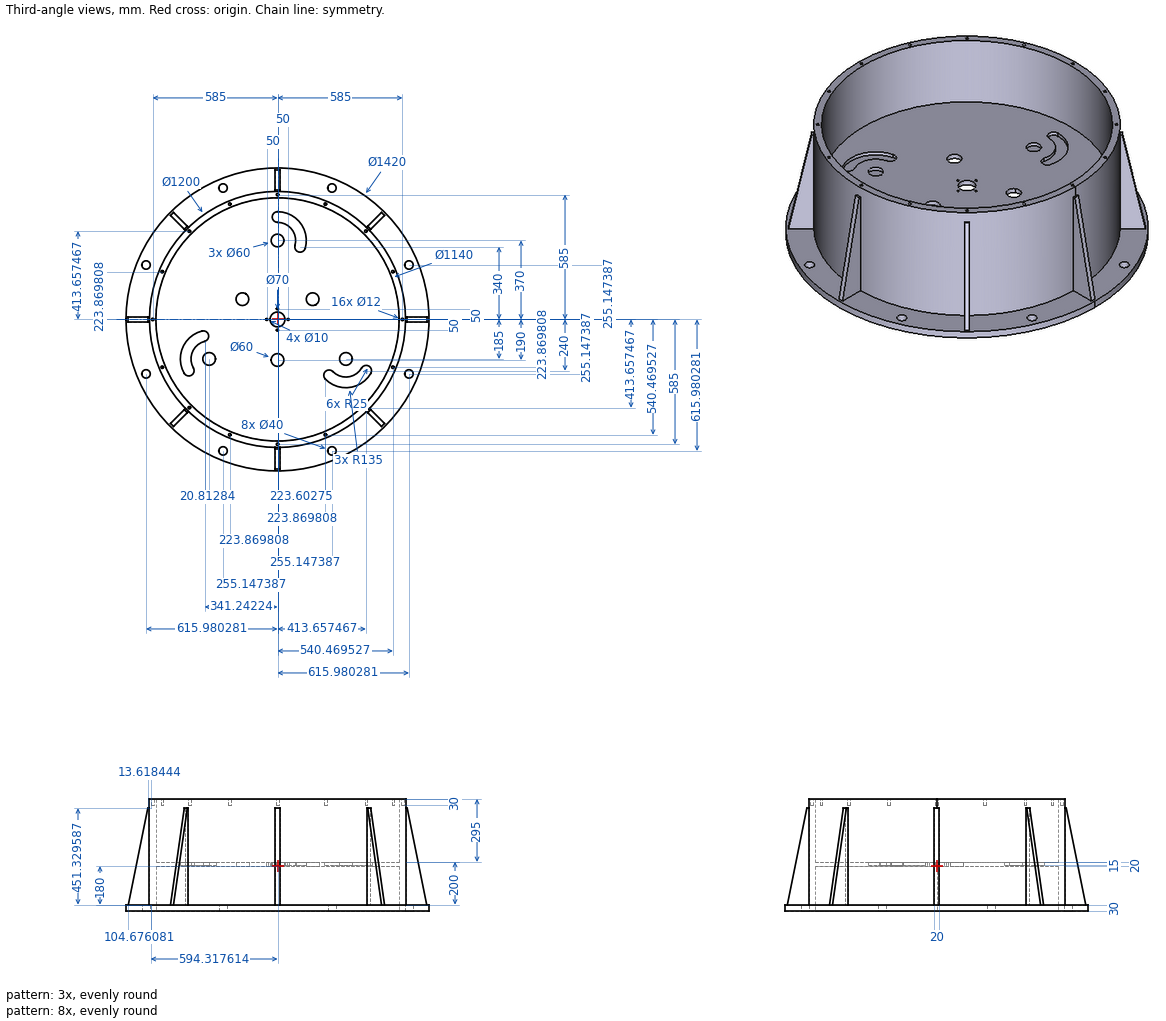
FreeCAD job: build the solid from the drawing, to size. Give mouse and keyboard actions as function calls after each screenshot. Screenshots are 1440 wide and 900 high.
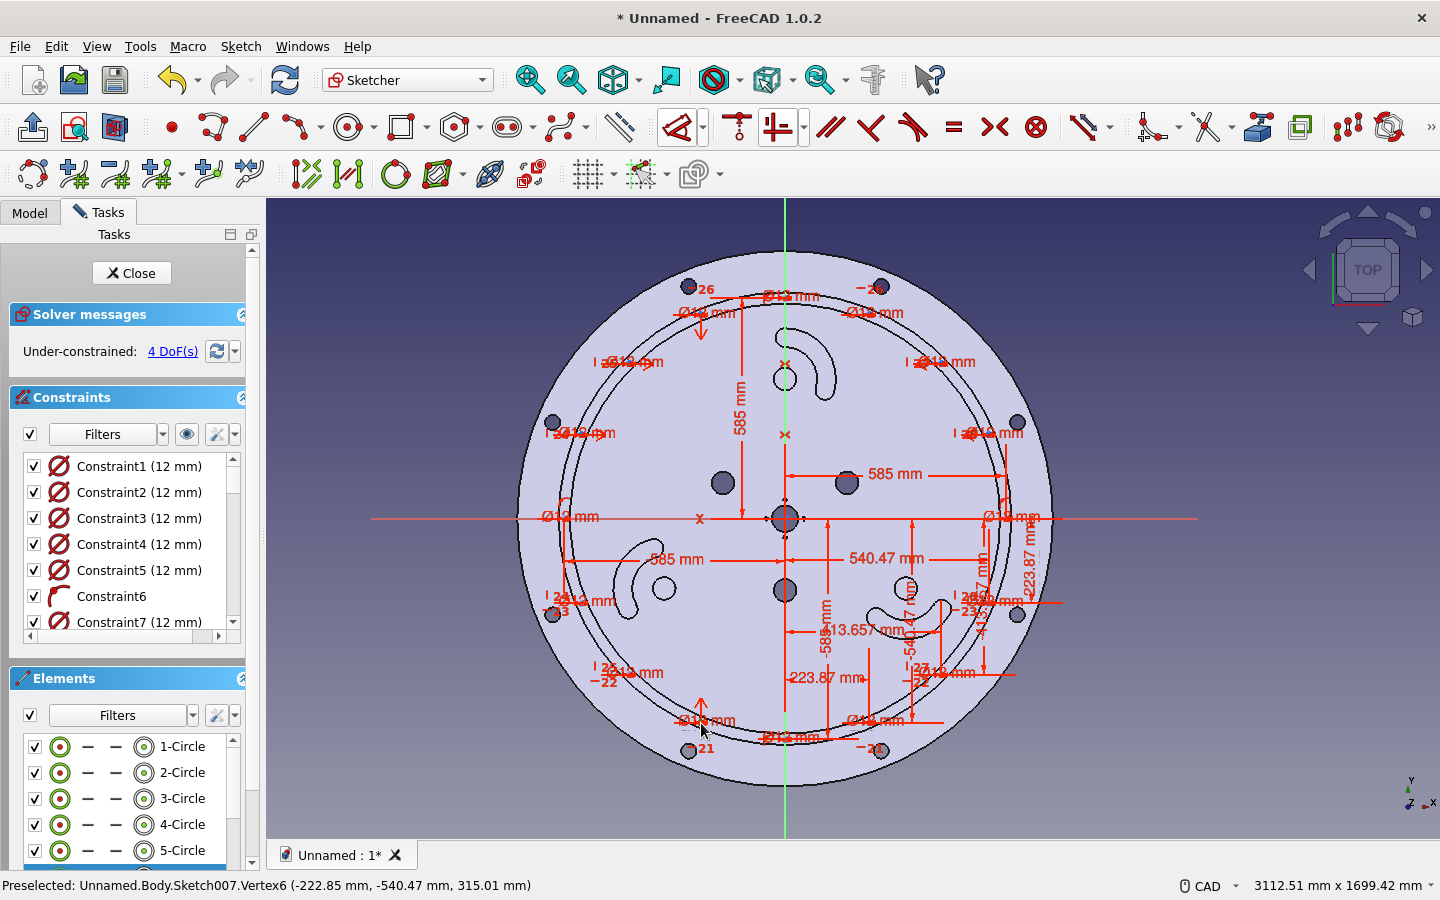
key(l)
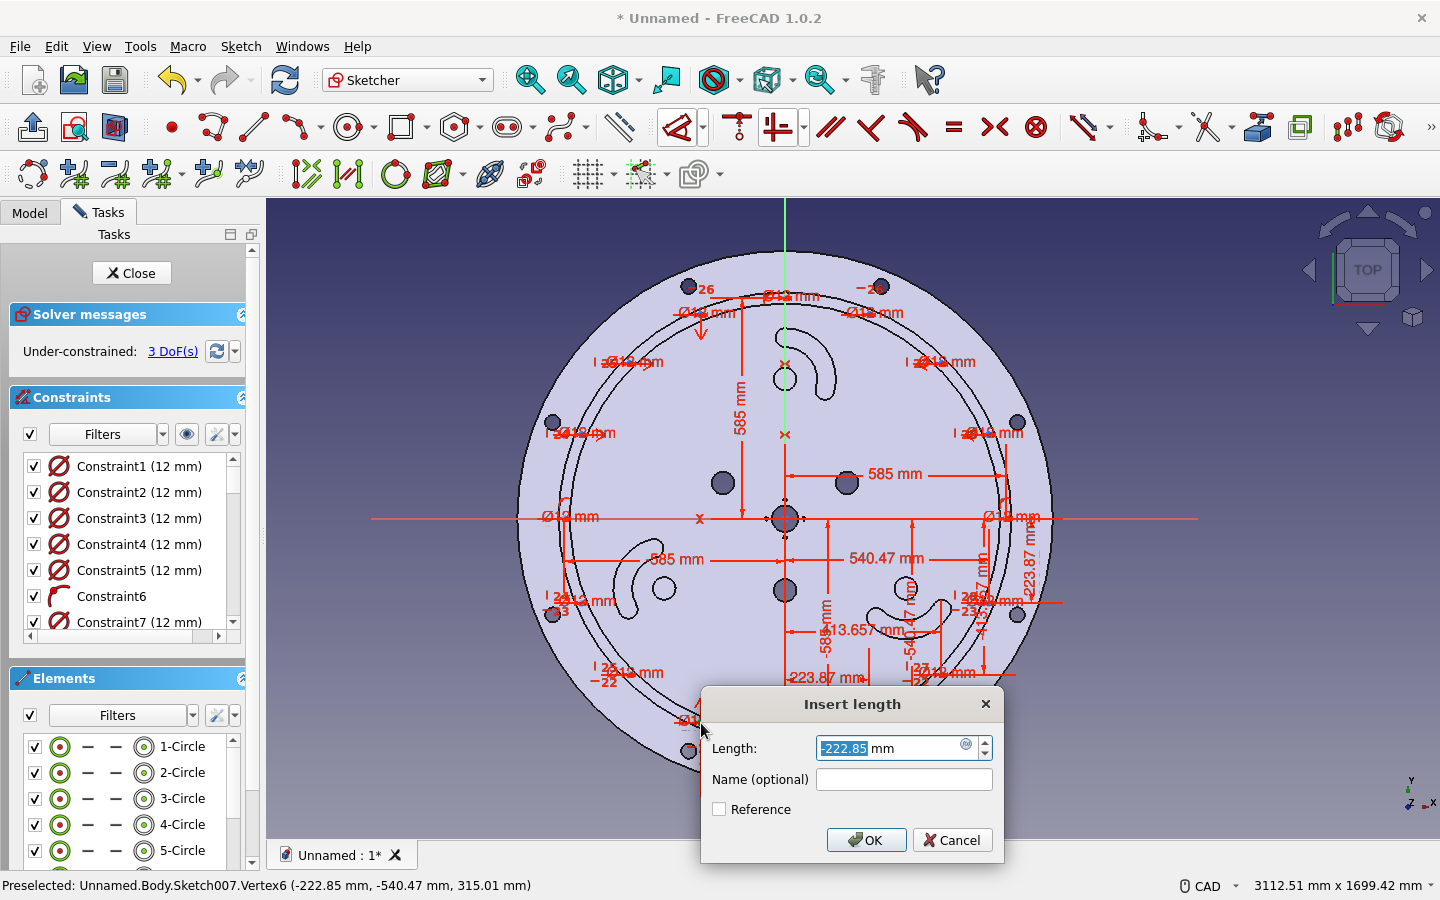
text(-223.869808)
key(Return)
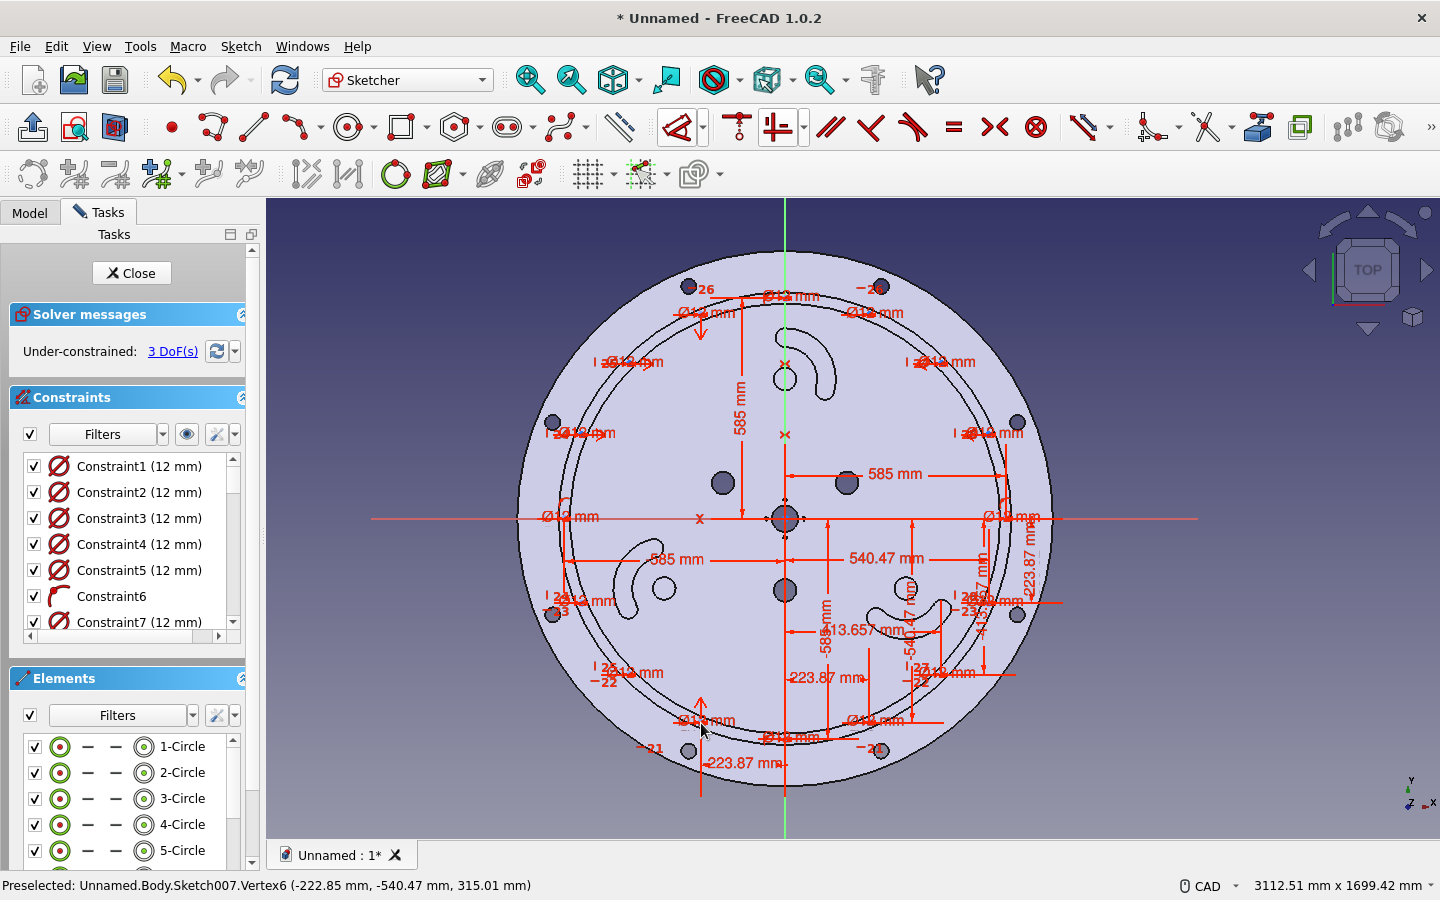
click(581, 435)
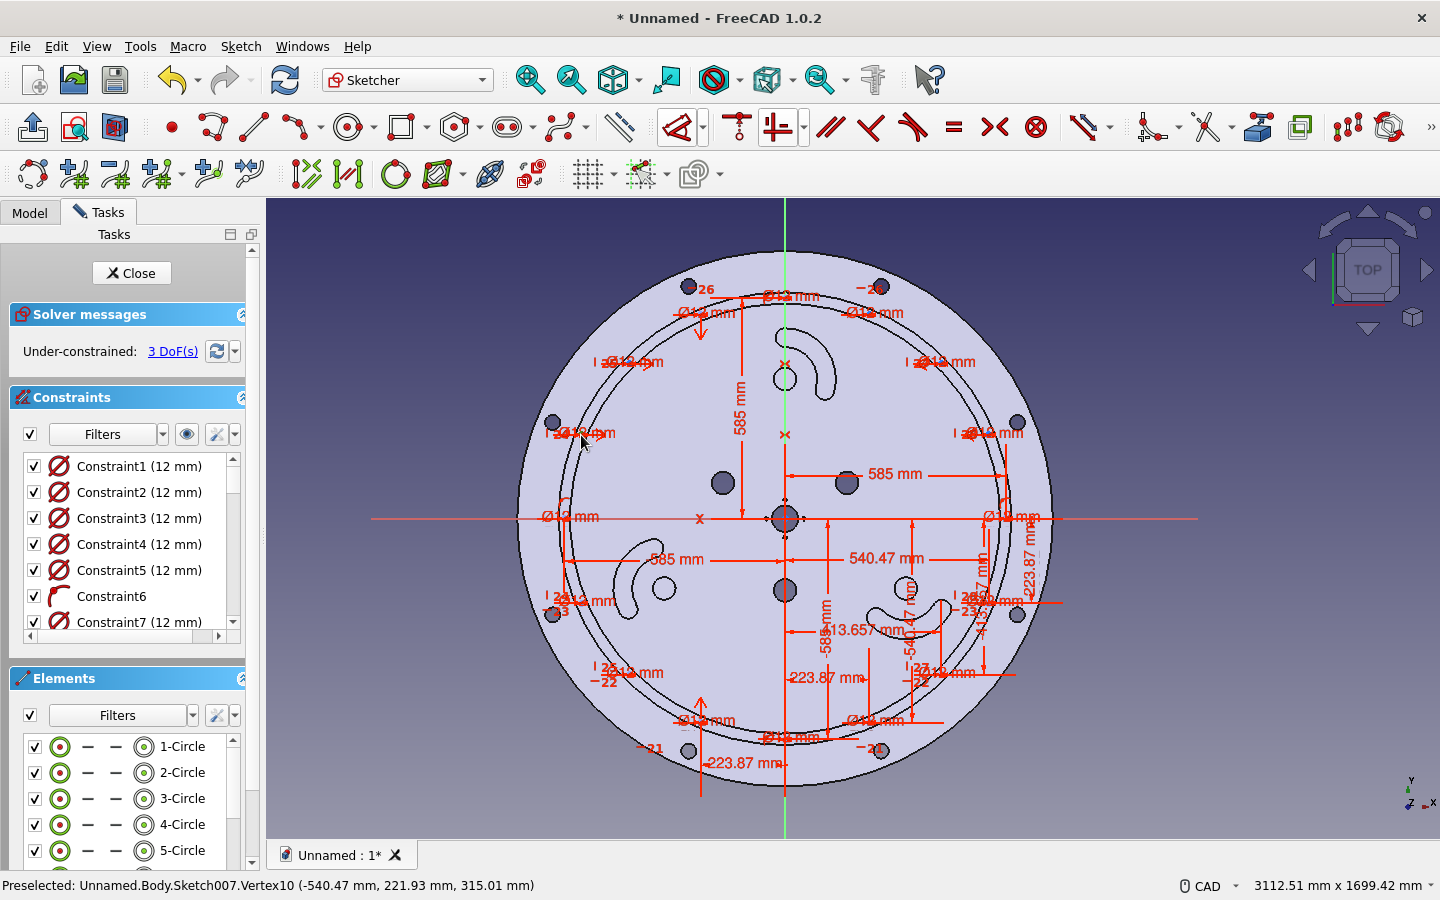
key(i)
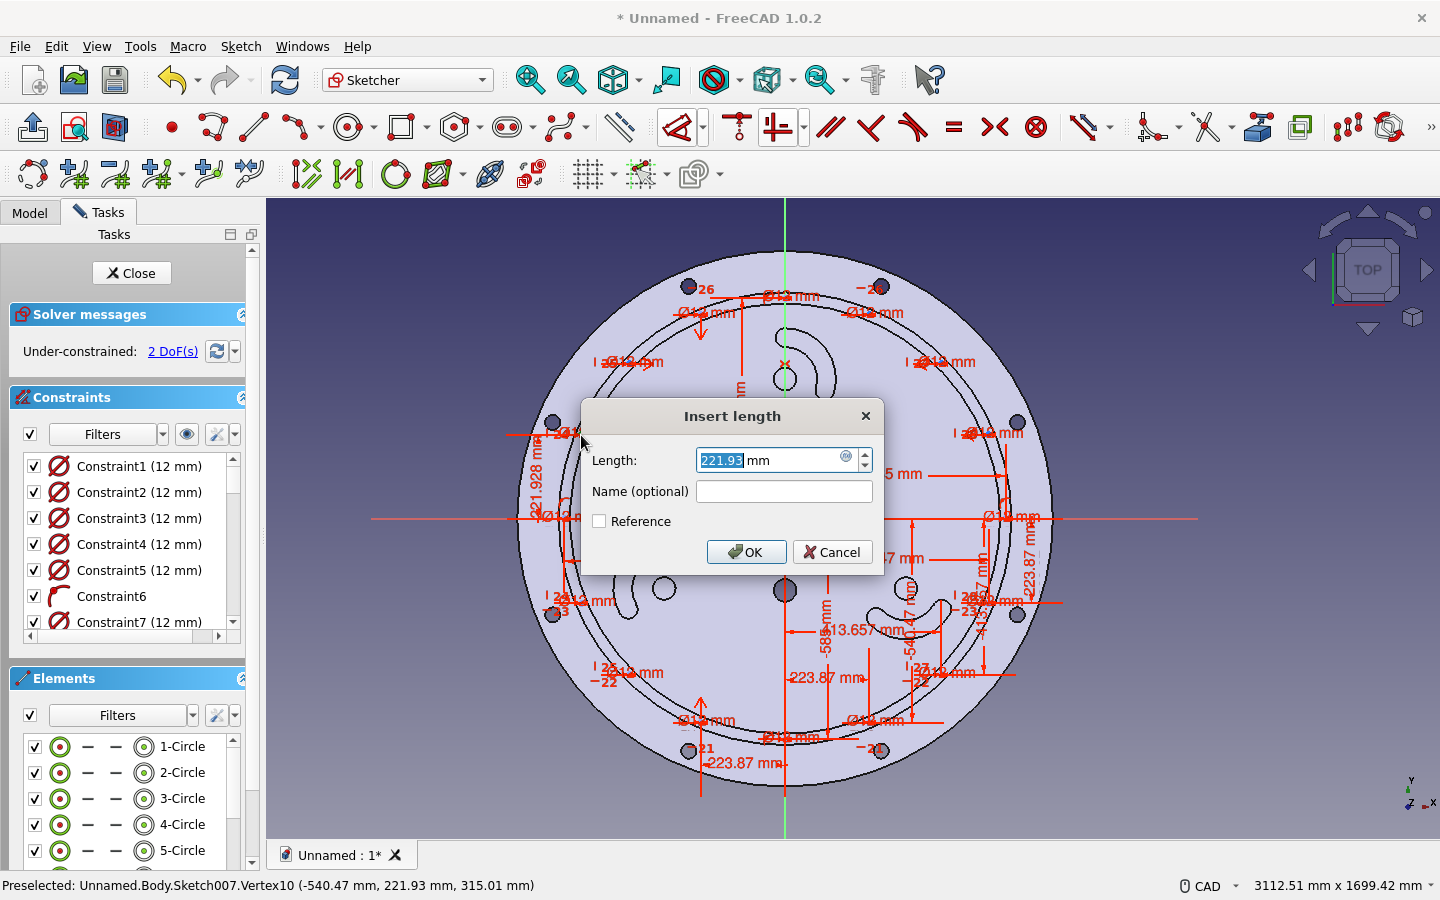
text(223.869808)
key(Return)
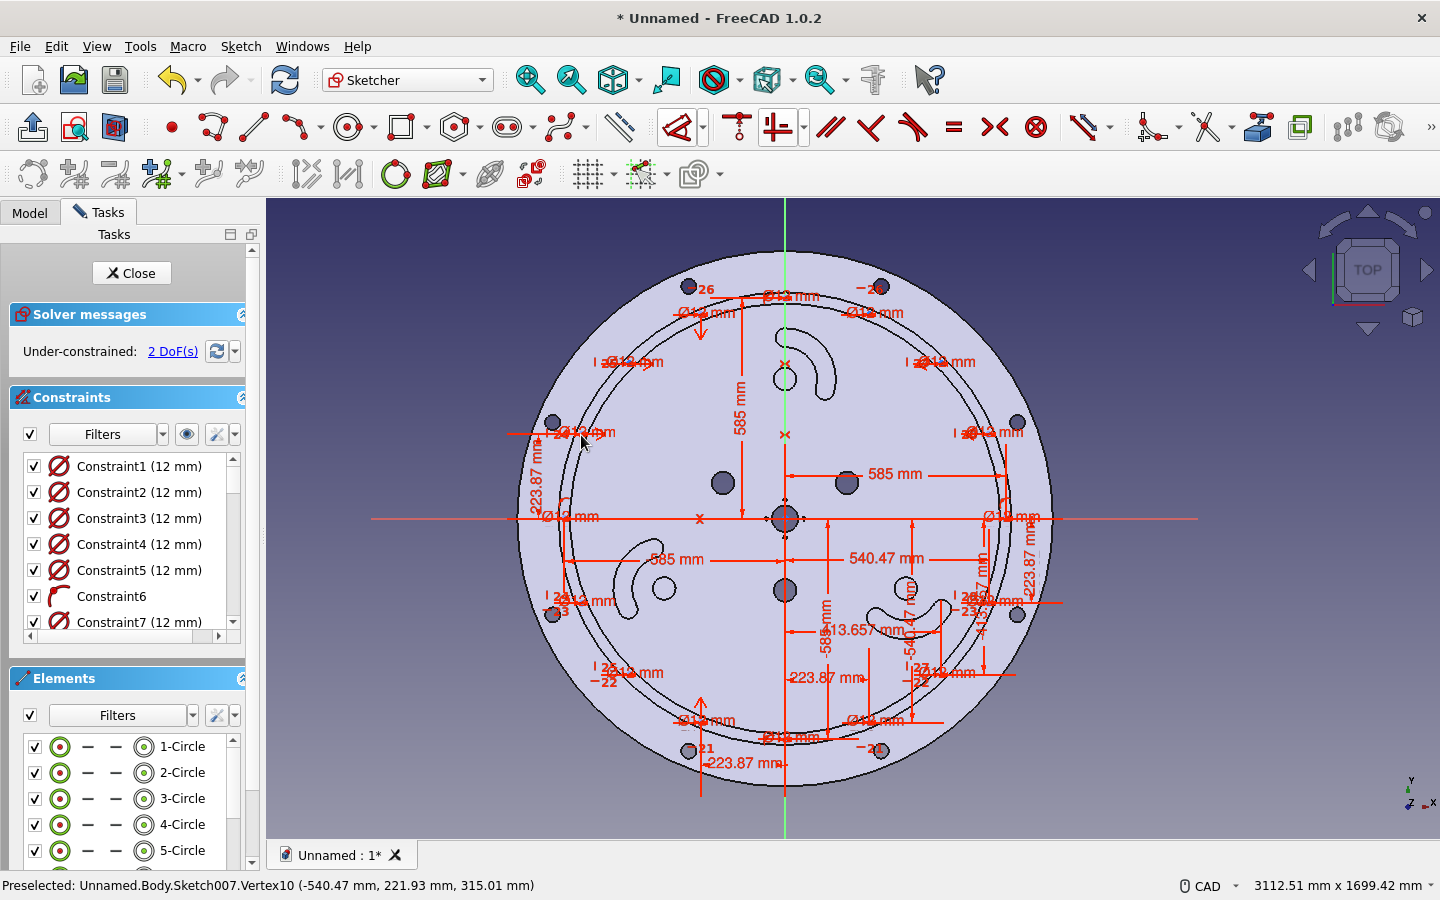
click(629, 364)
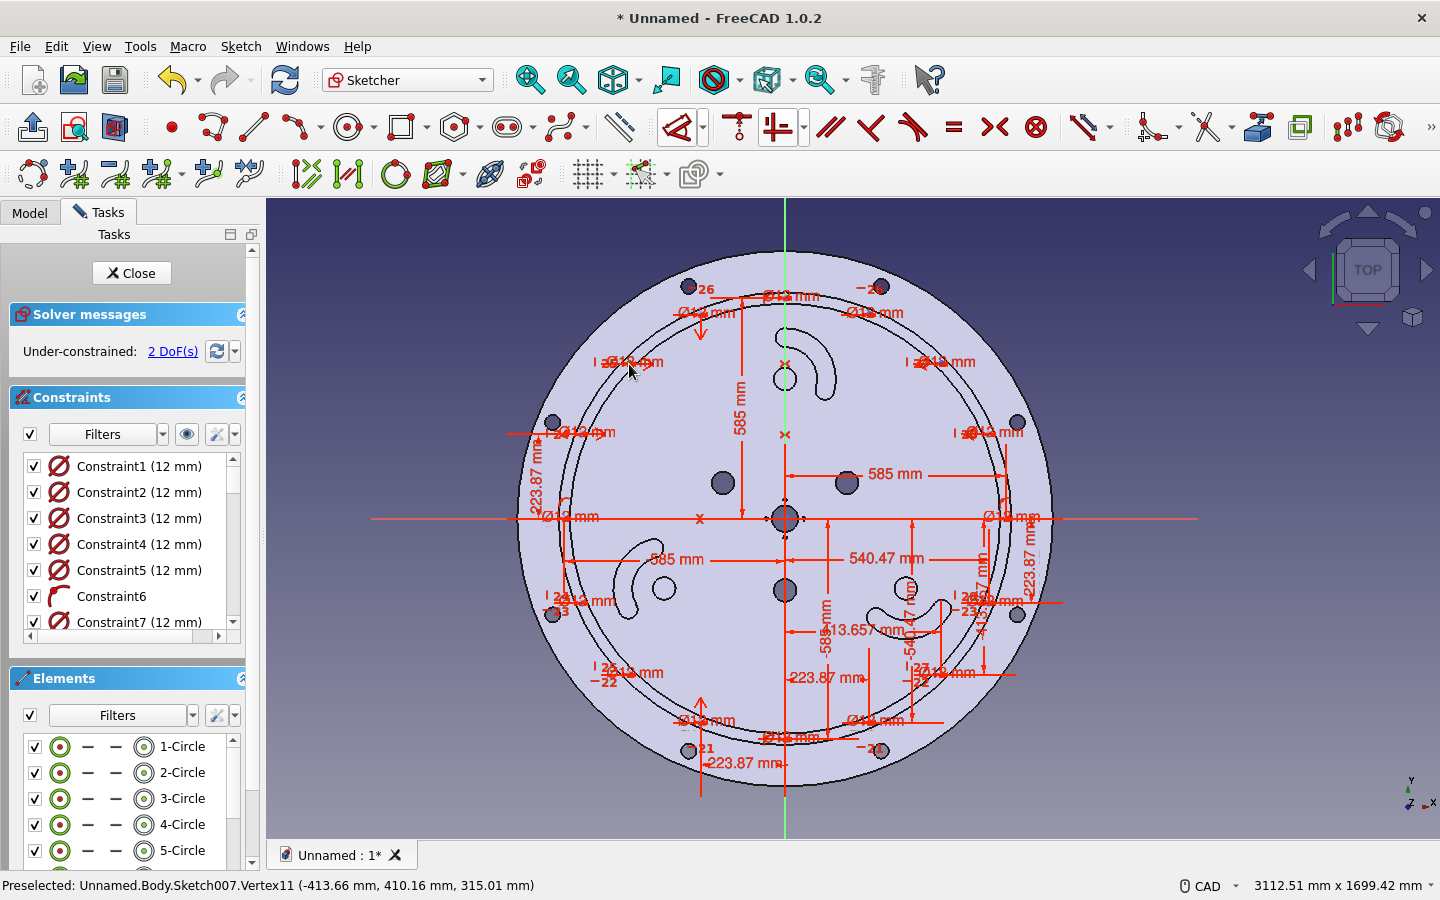
key(i)